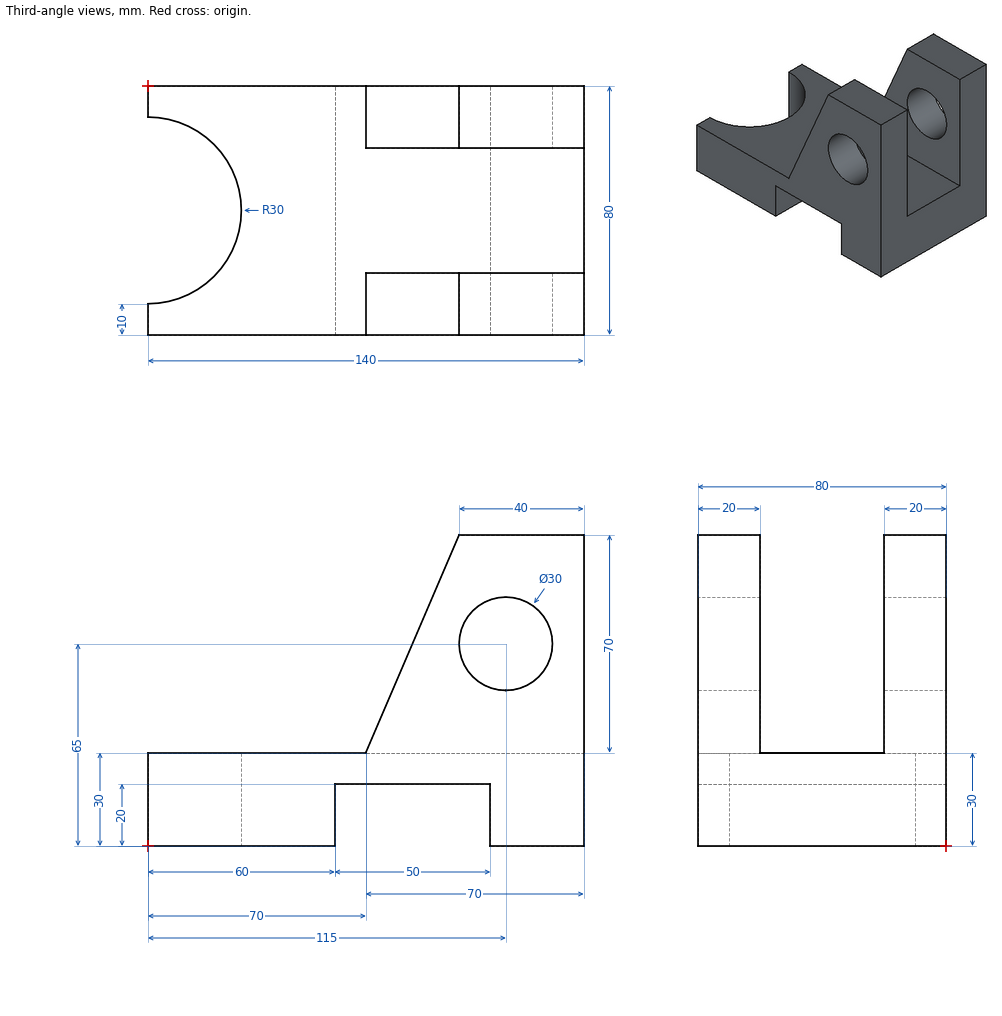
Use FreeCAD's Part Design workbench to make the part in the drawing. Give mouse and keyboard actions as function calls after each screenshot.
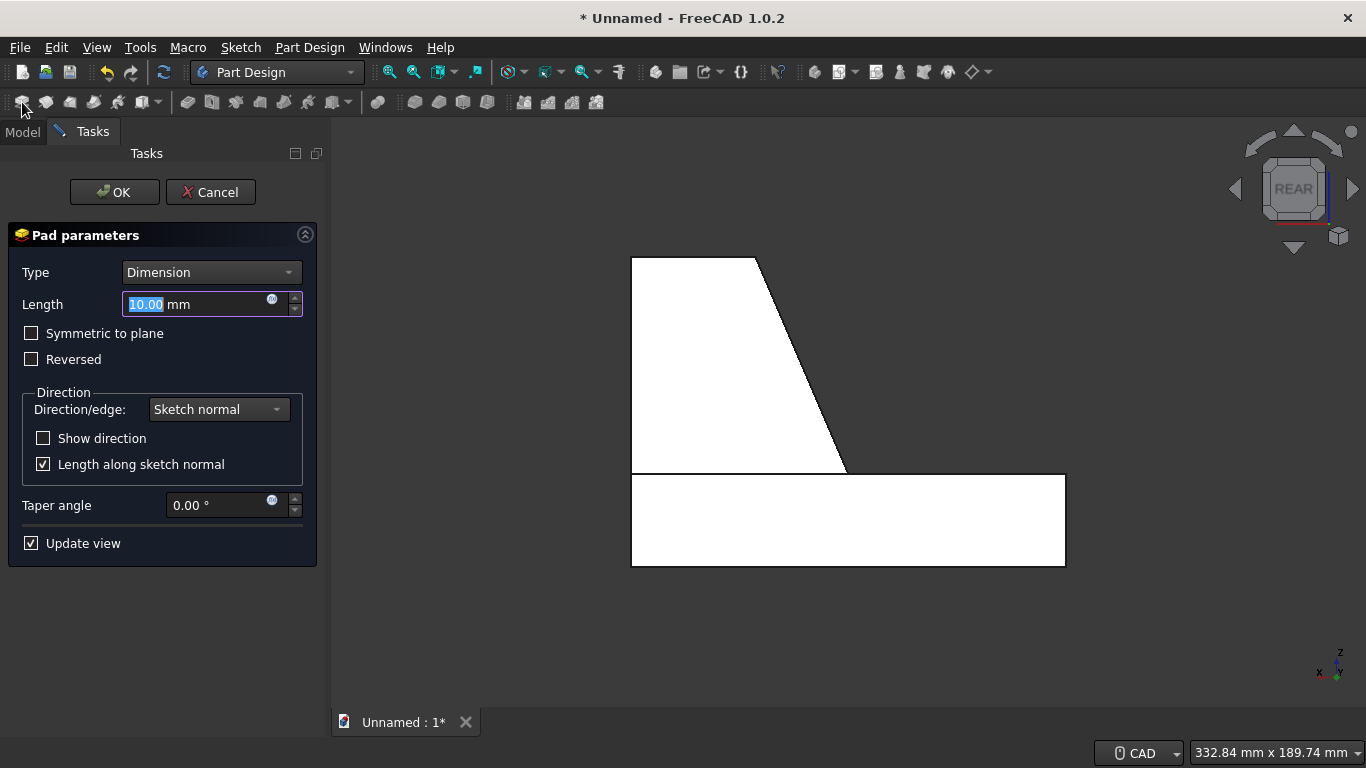
text(20)
key(Tab)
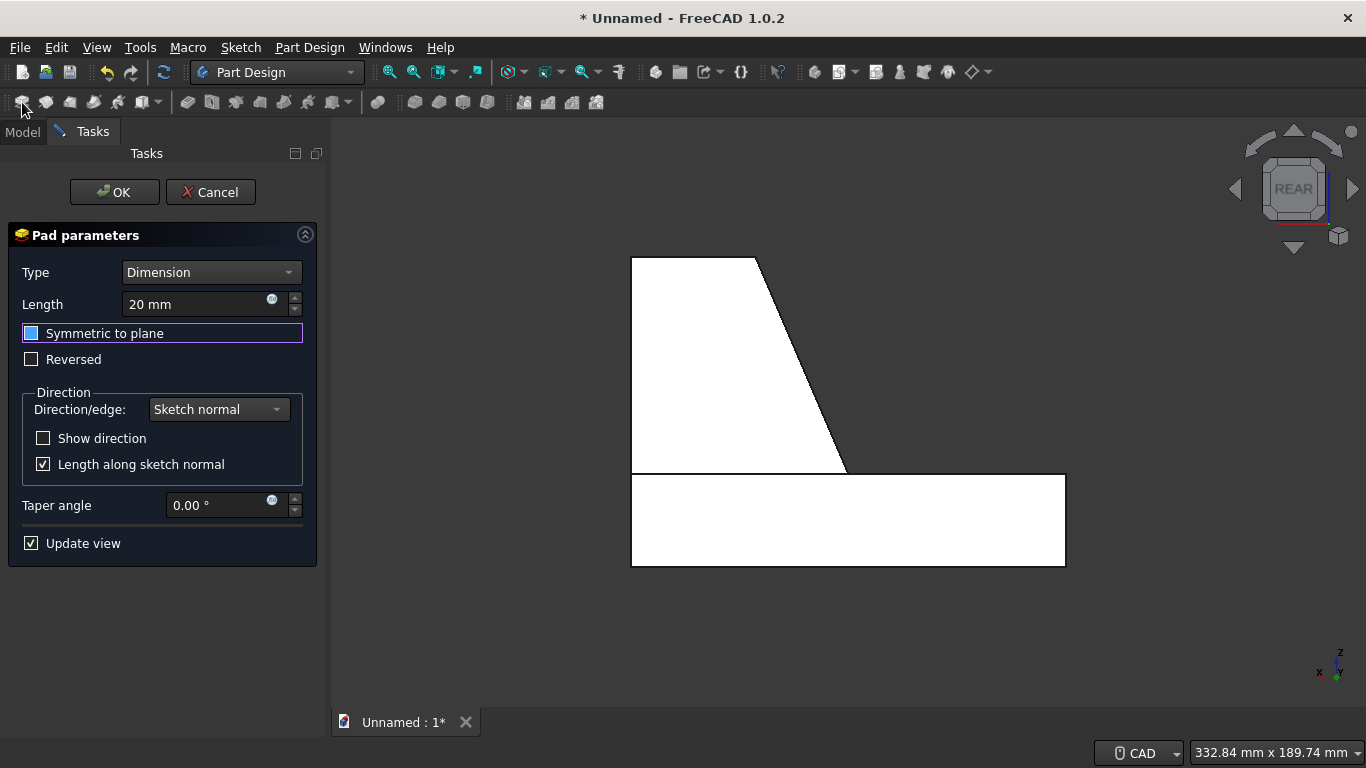
click(30, 359)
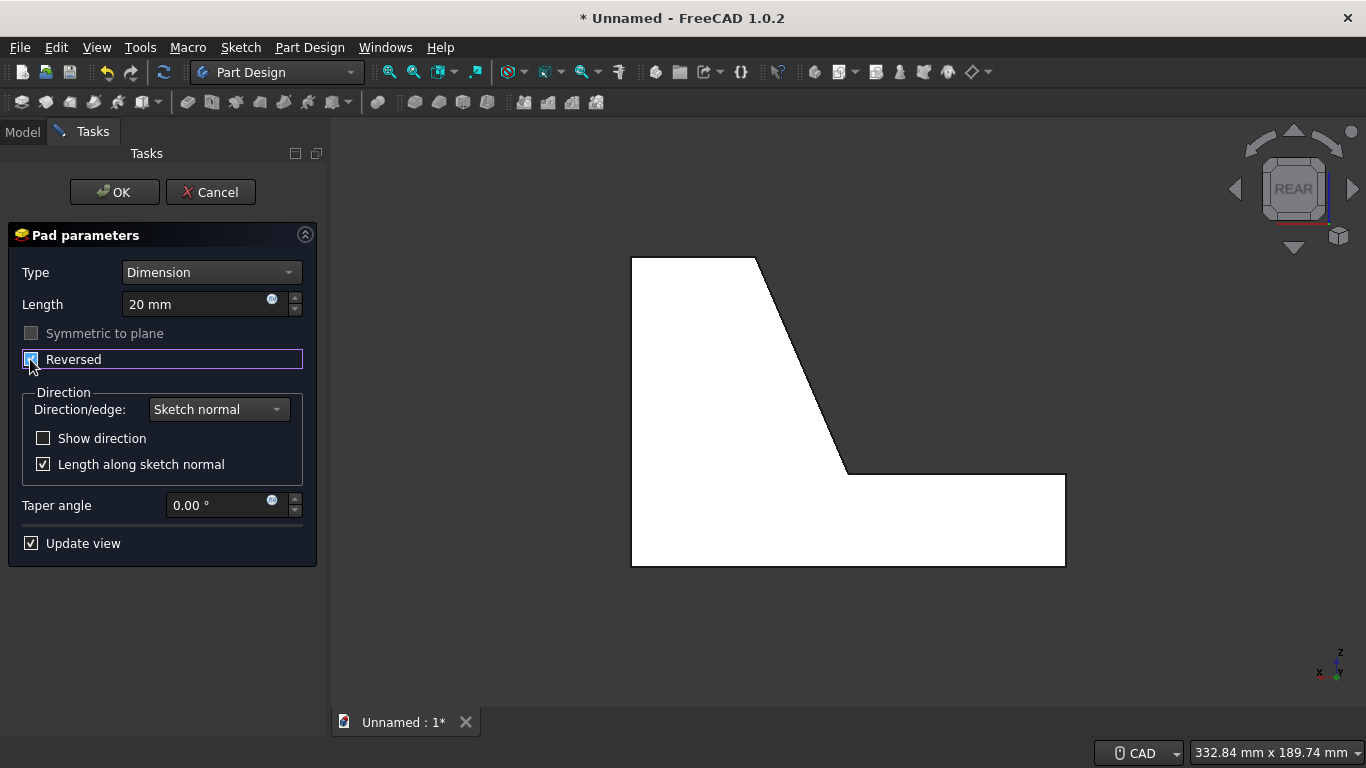
click(115, 192)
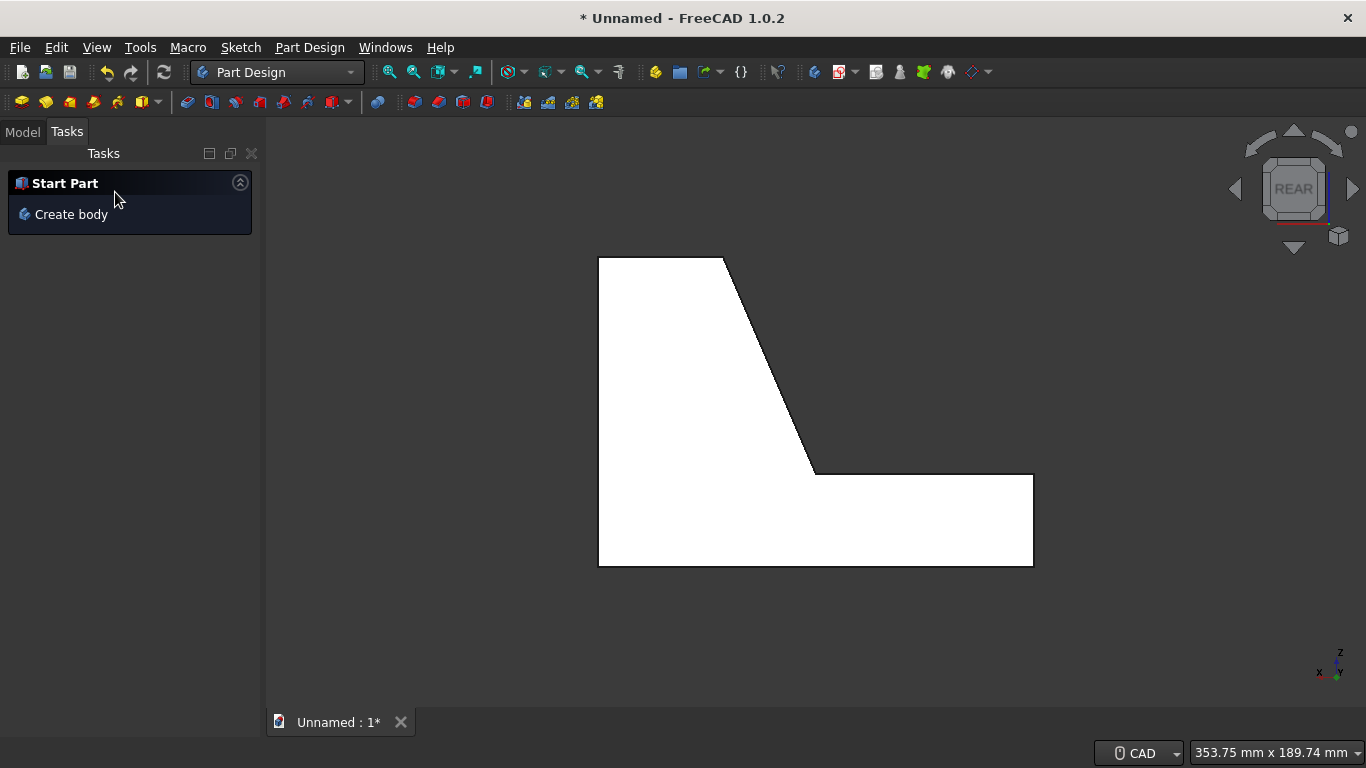
key(0)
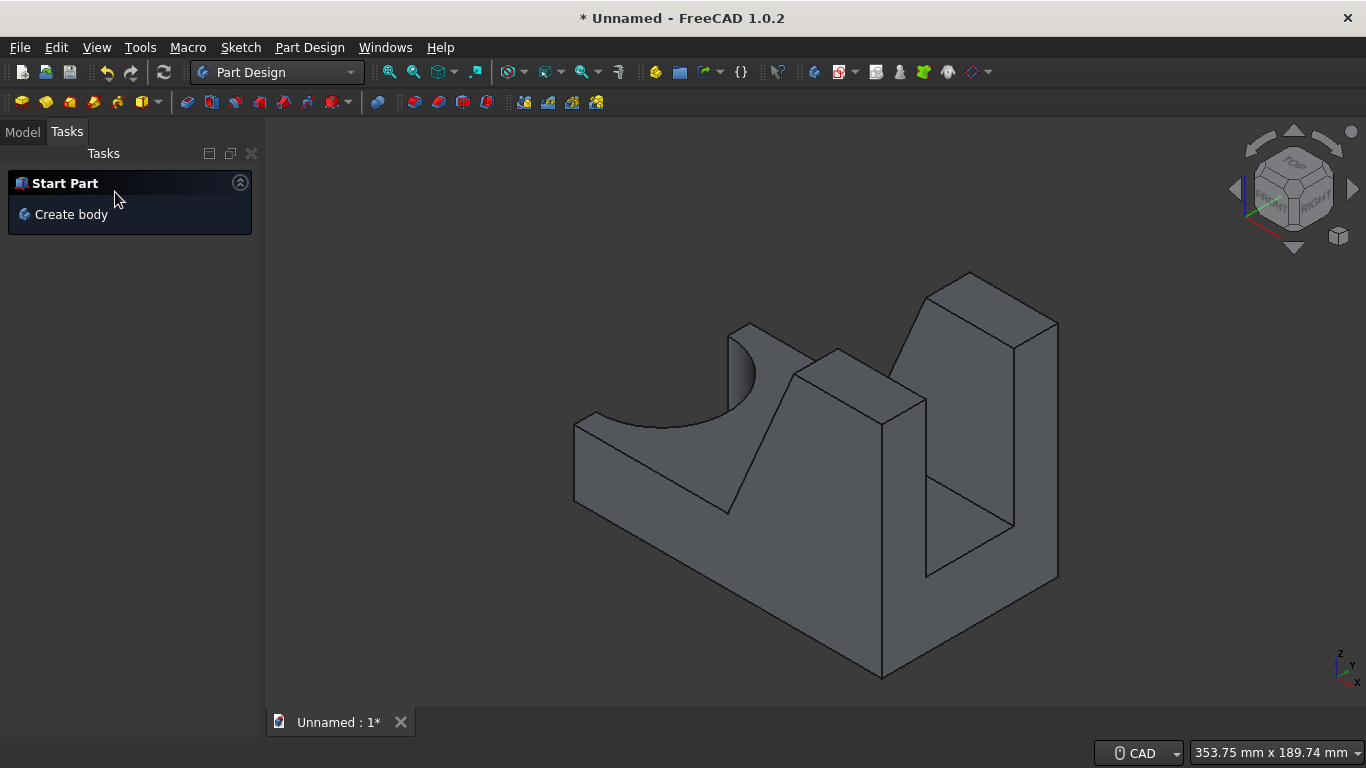
click(816, 549)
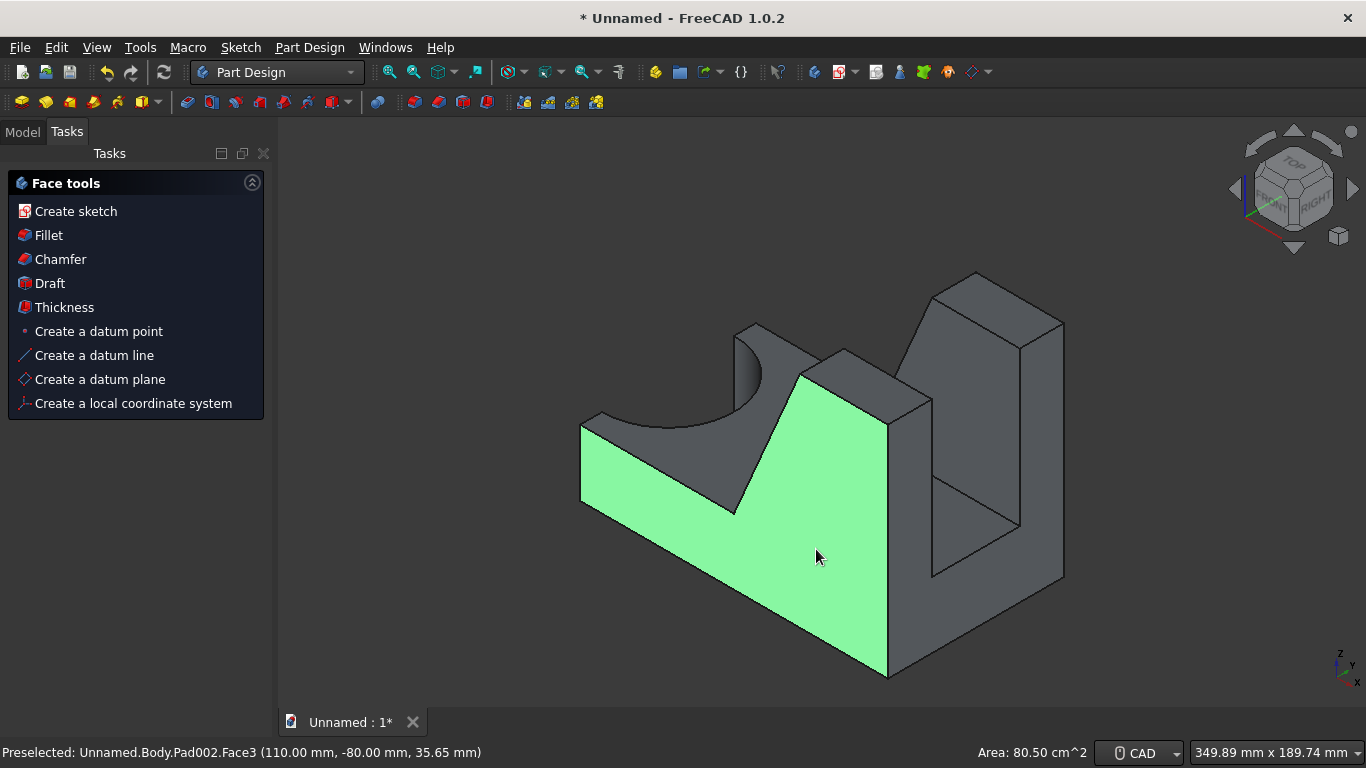
click(840, 72)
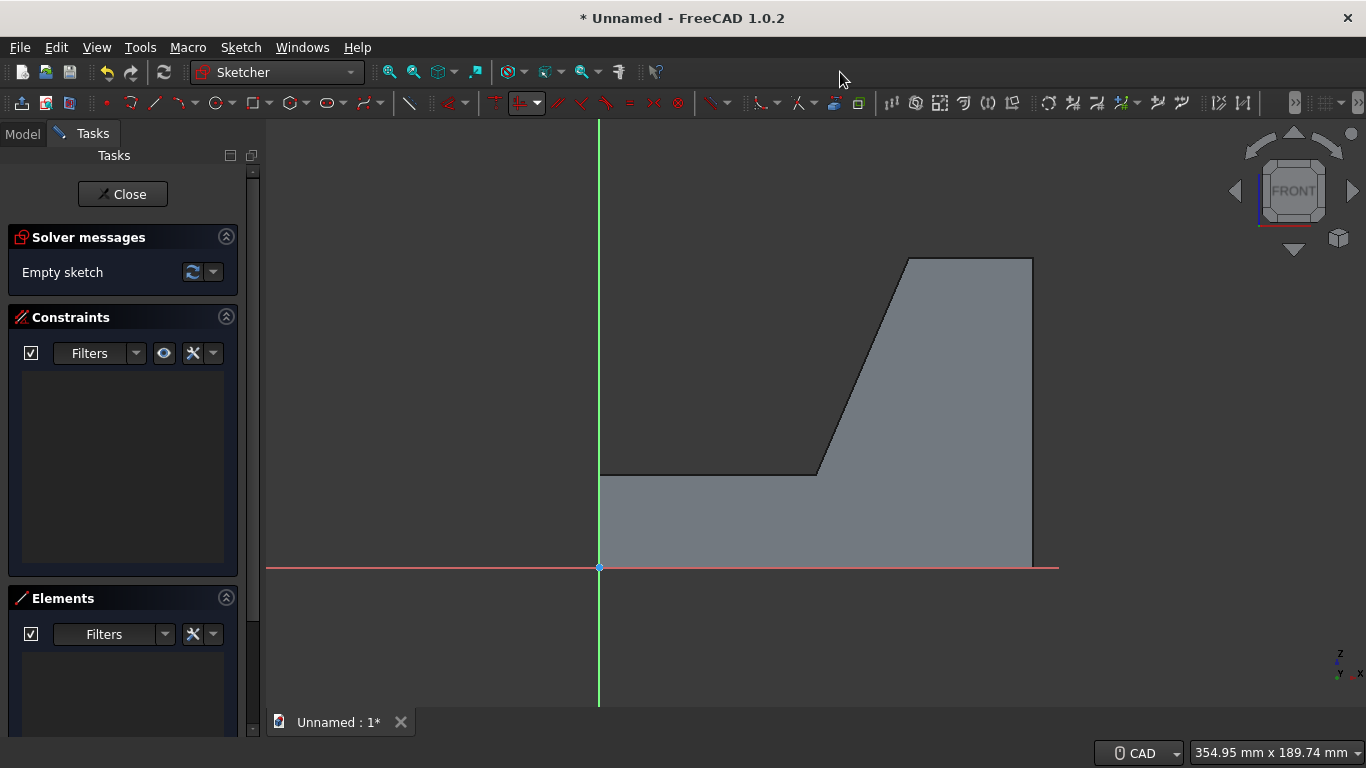
scroll(1024, 351, up, 7)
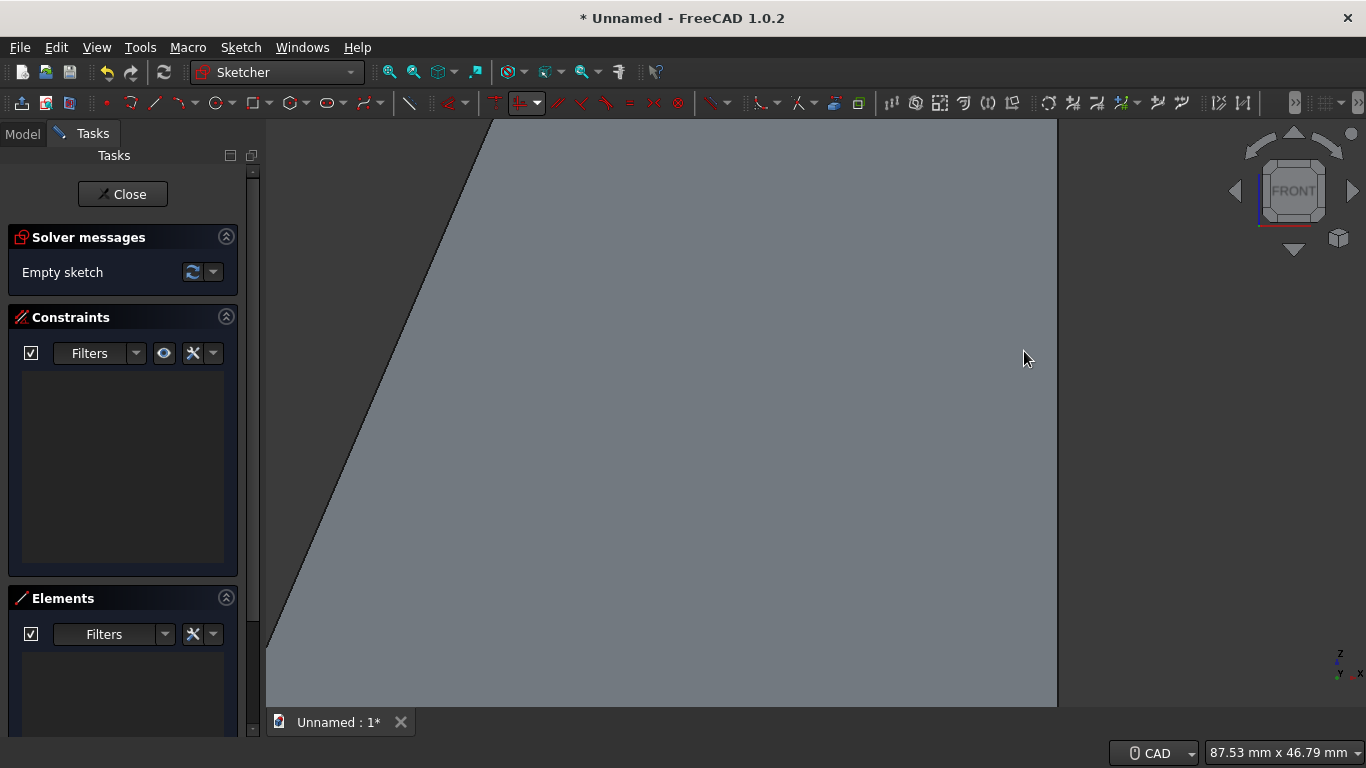
click(216, 104)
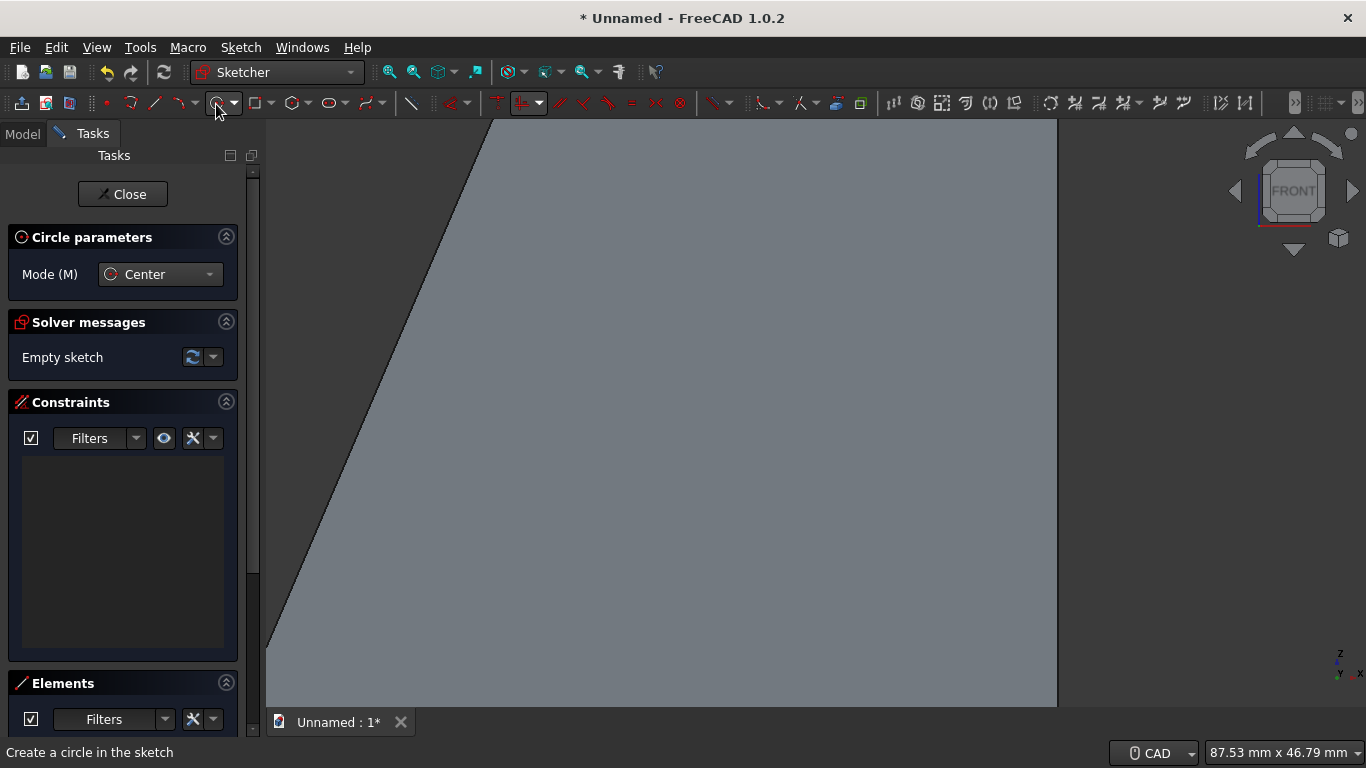
click(744, 413)
move(877, 279)